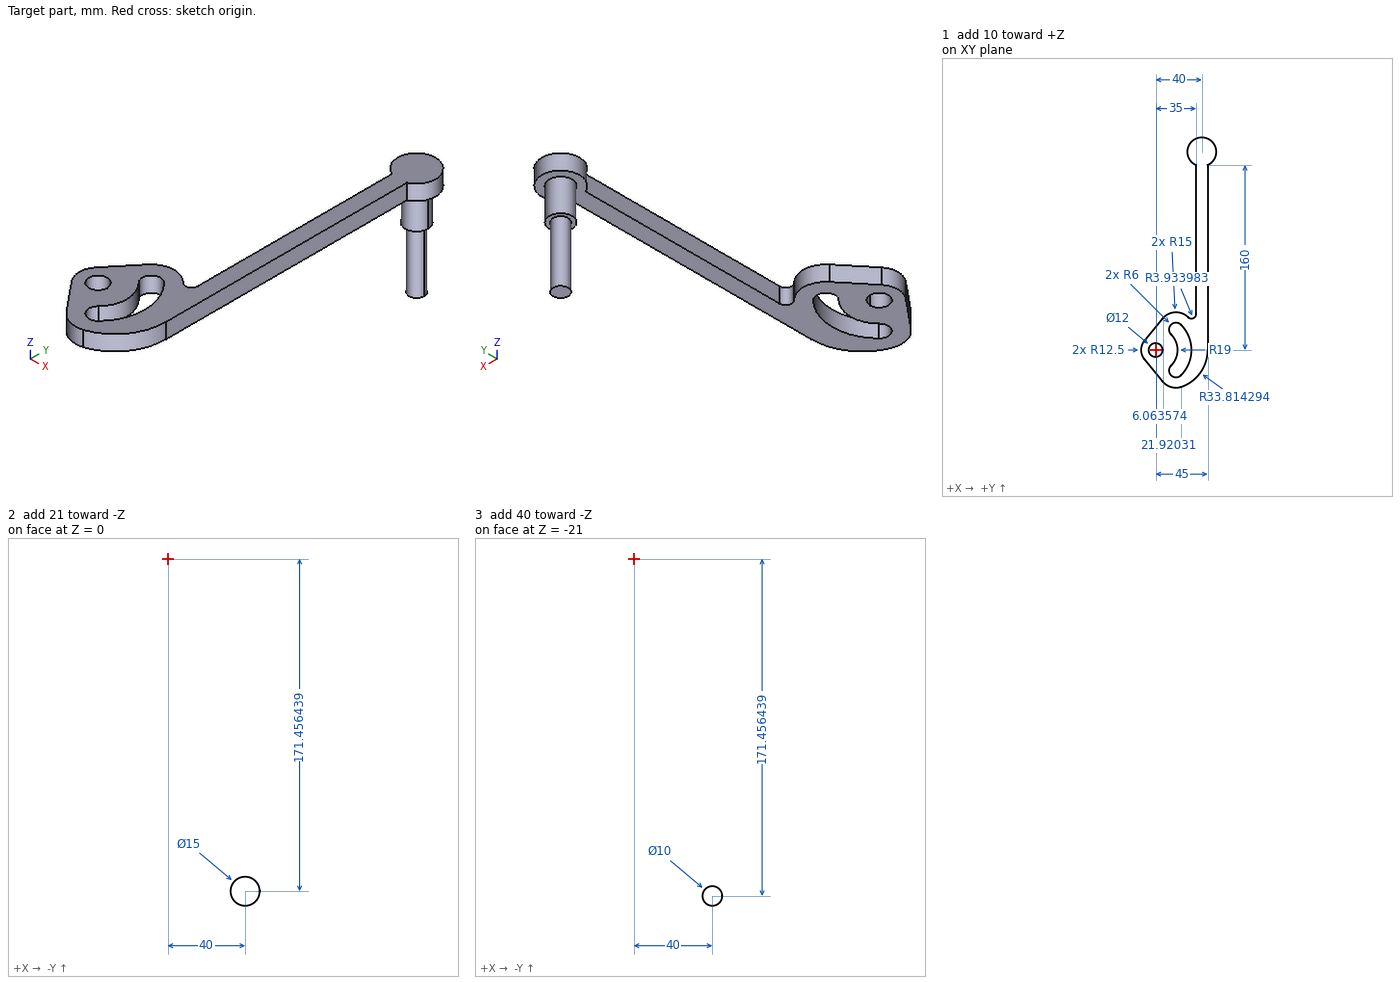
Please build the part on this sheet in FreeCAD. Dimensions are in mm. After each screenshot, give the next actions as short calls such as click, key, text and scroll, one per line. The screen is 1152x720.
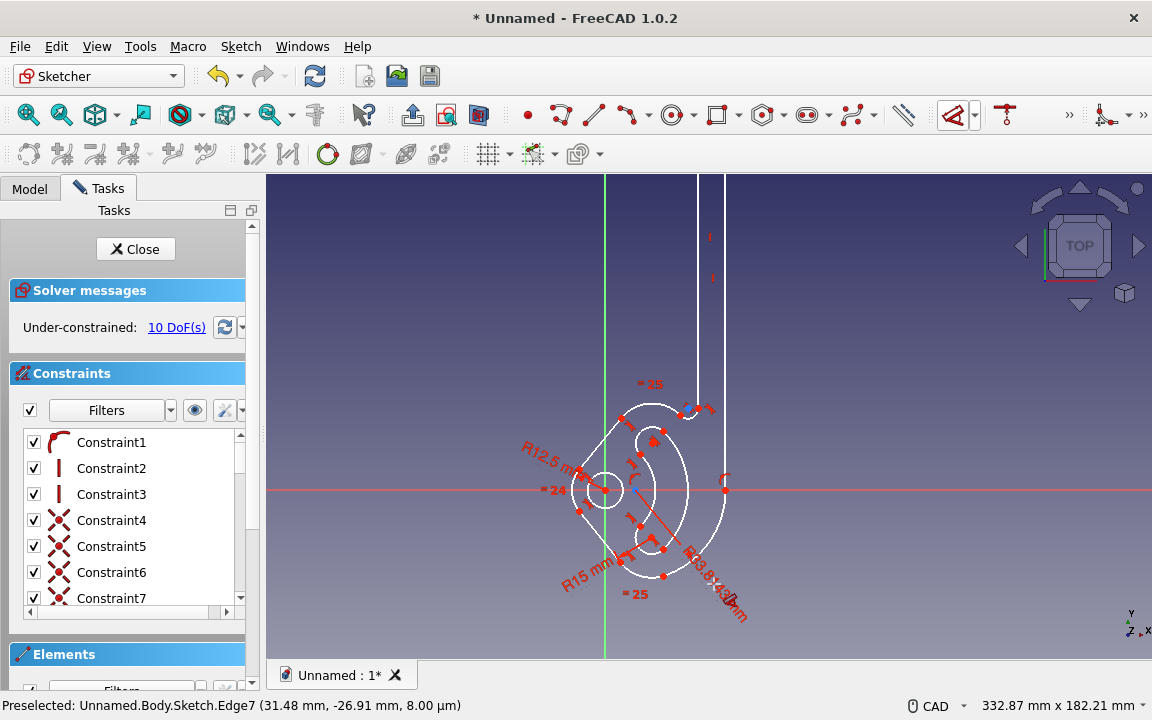
scroll(692, 418, up, 7)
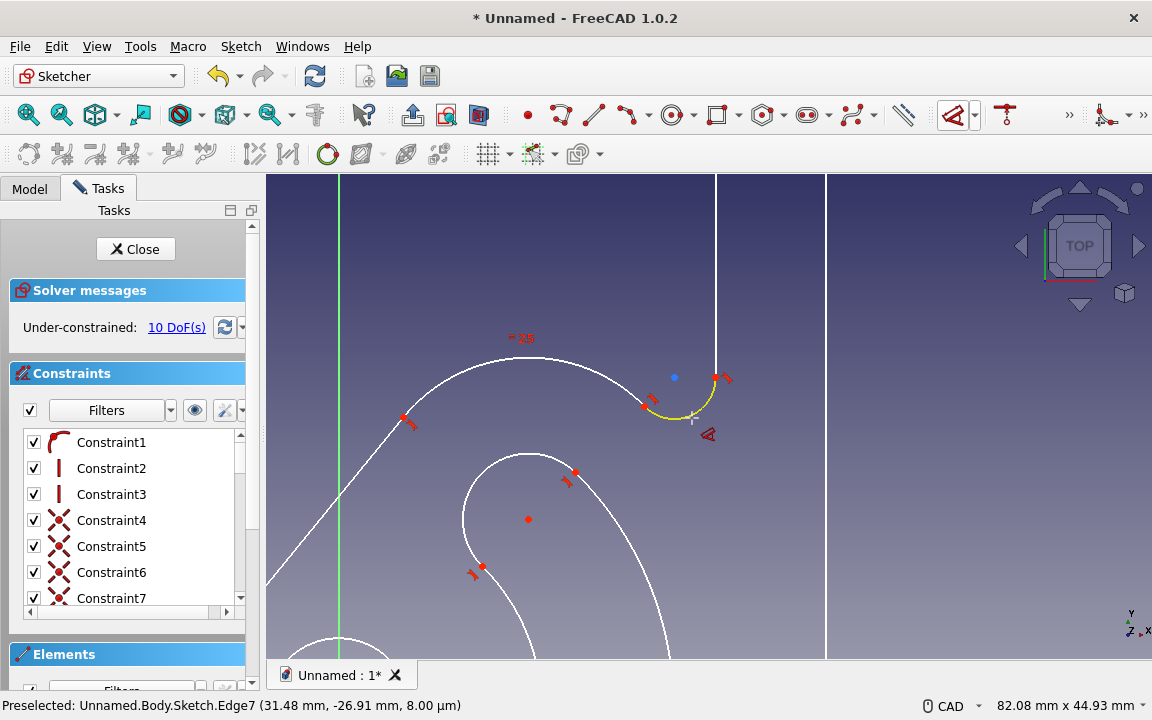
click(690, 416)
click(702, 446)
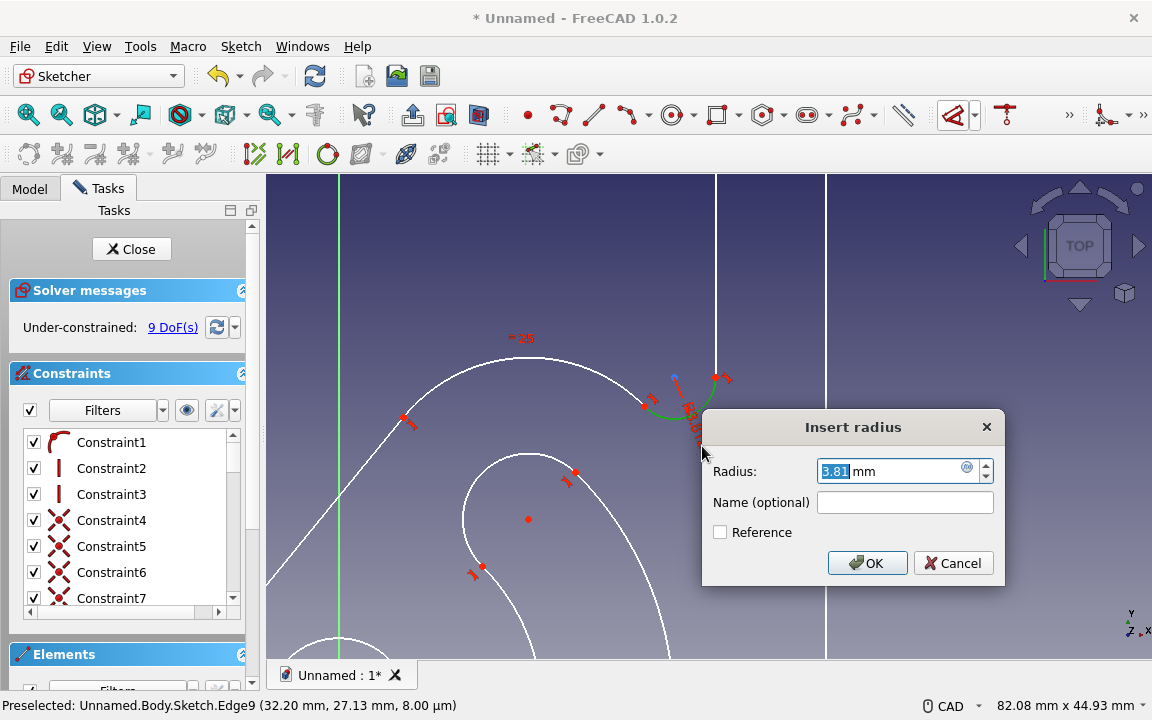
text(3.933983)
key(Return)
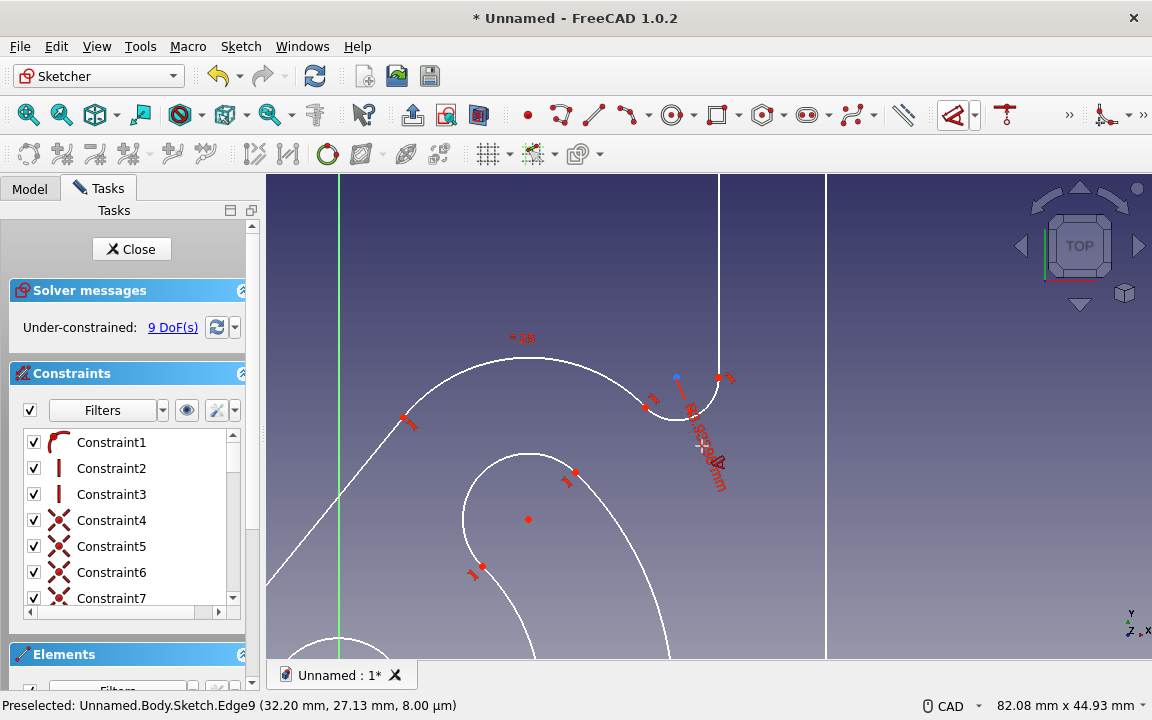
scroll(660, 499, down, 10)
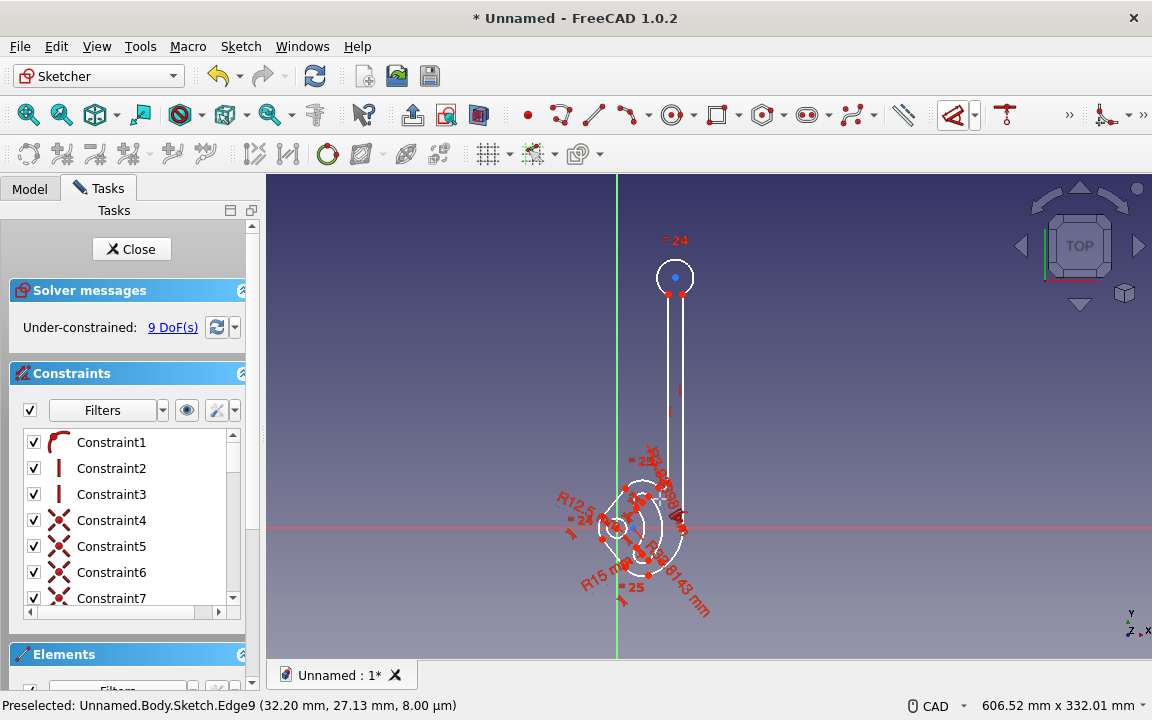
scroll(641, 516, up, 3)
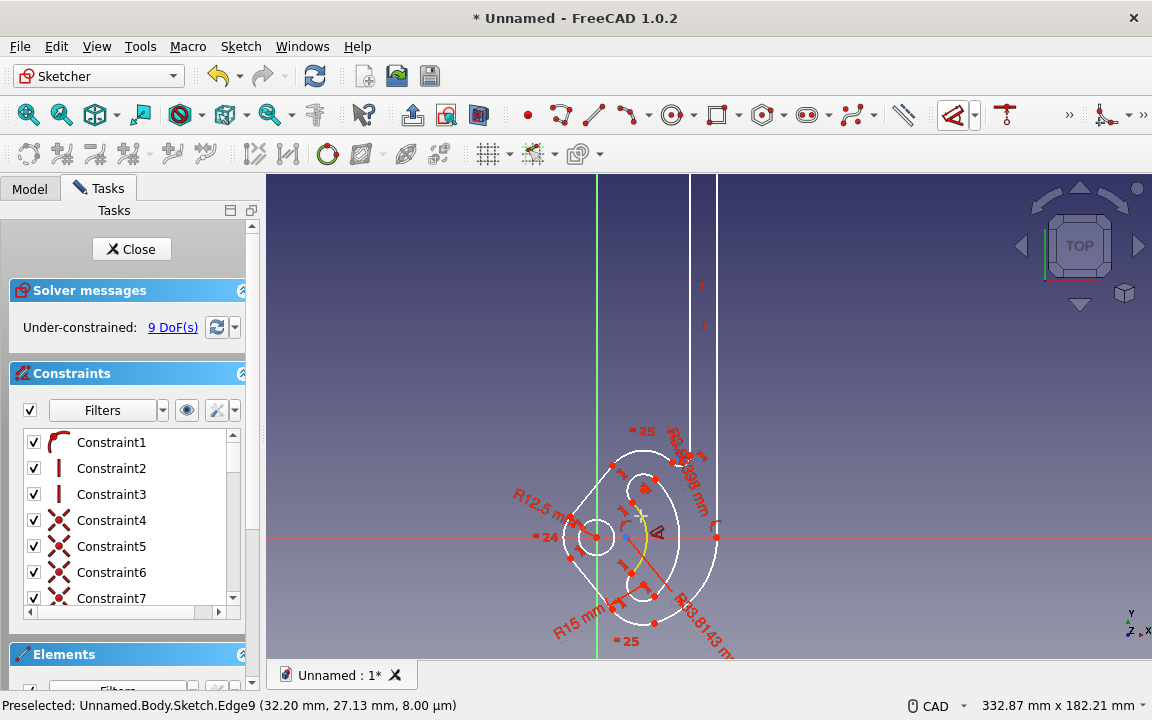
click(641, 515)
click(560, 465)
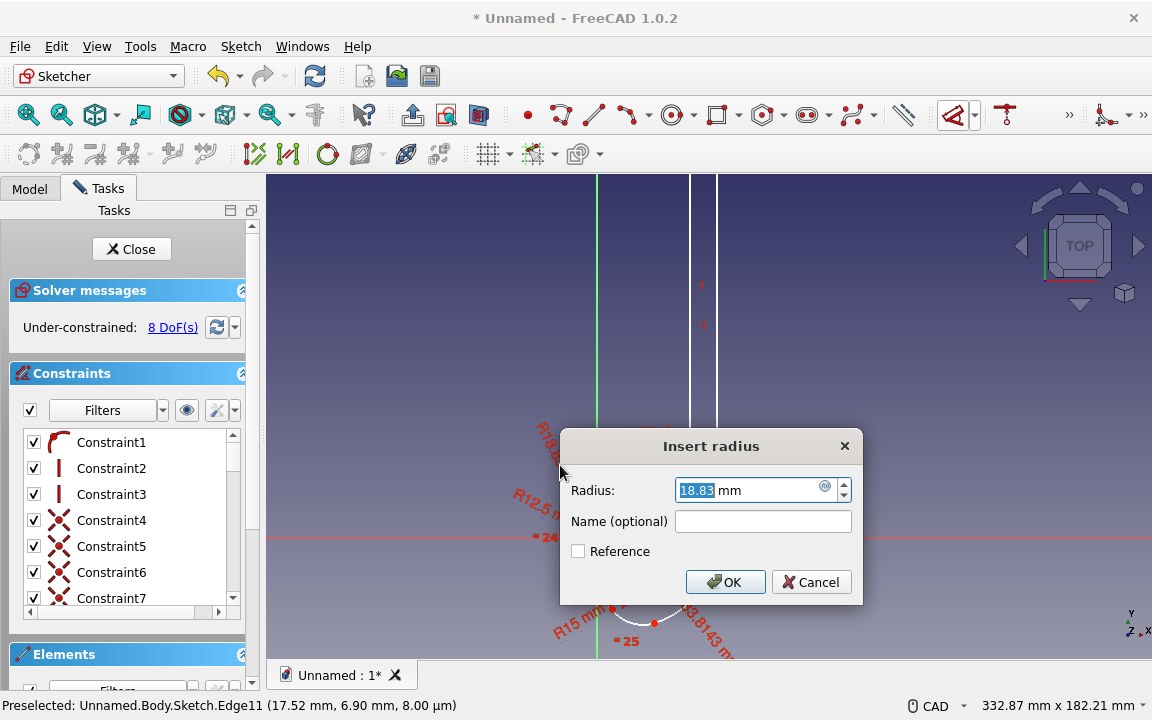
text(19)
key(Return)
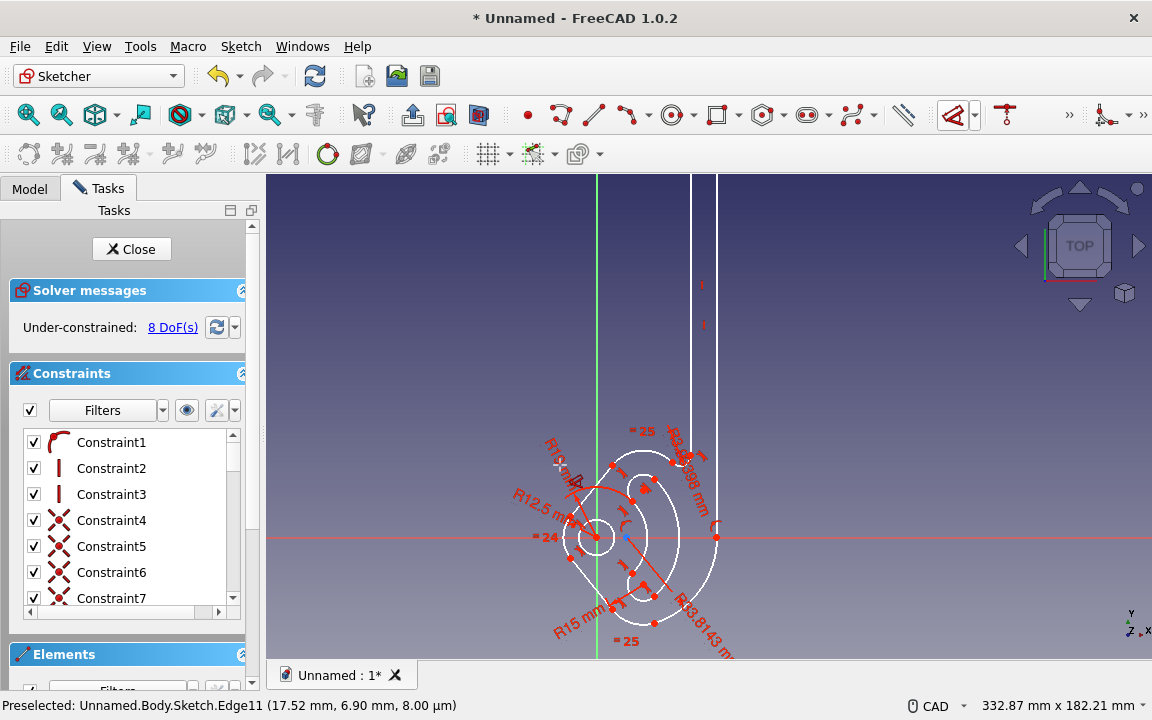
scroll(641, 475, up, 5)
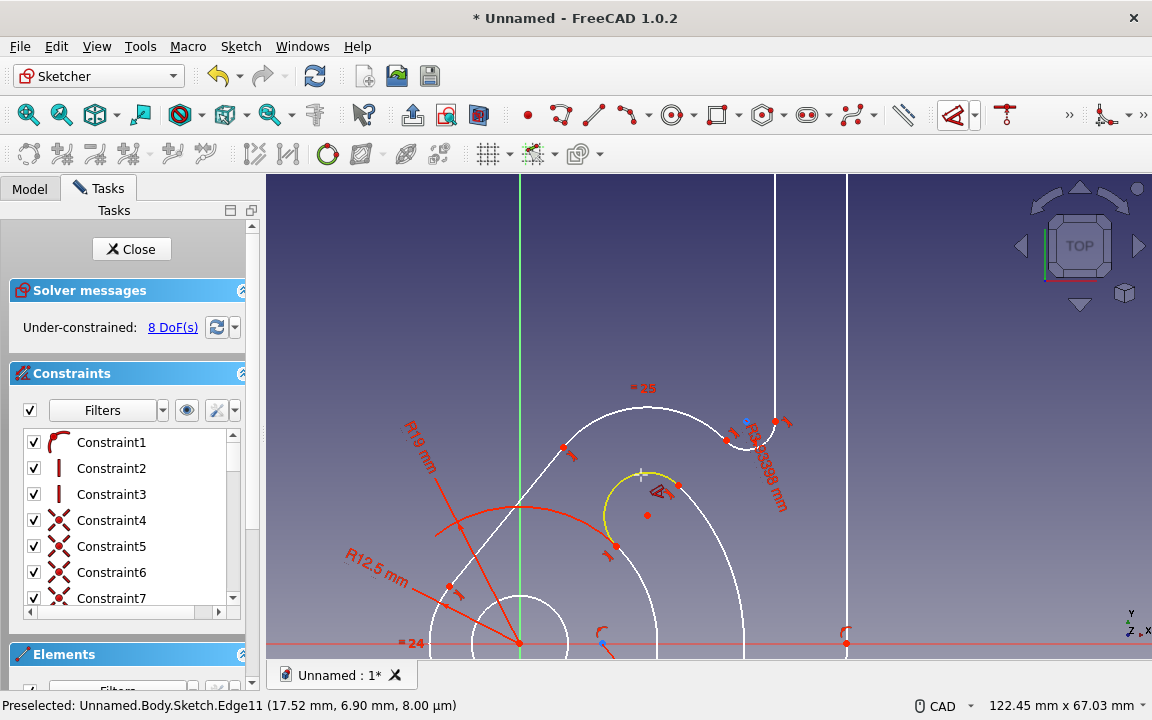
click(641, 473)
click(636, 441)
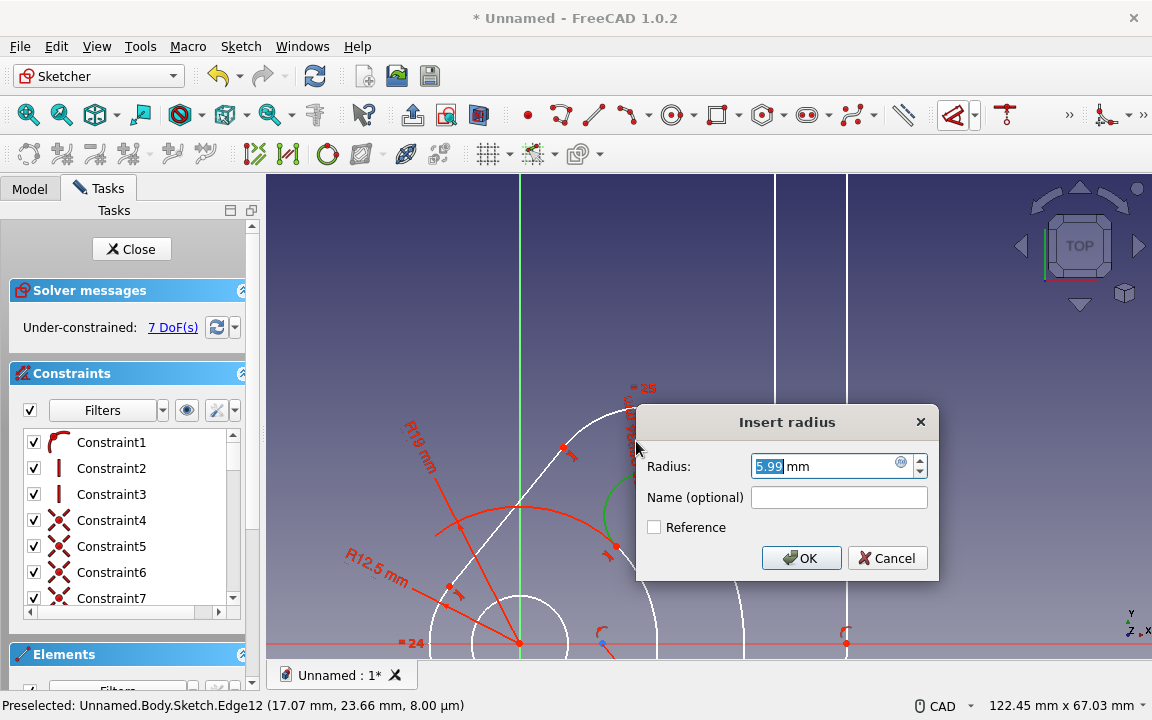
text(6)
key(Return)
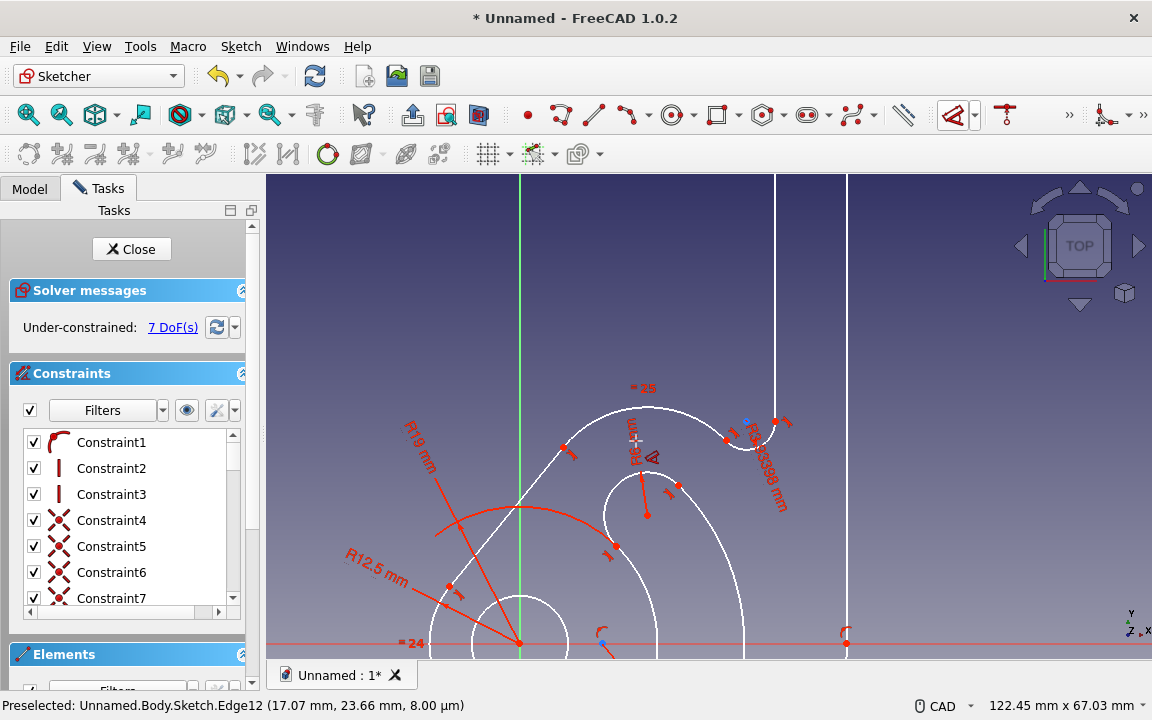
click(554, 610)
click(577, 587)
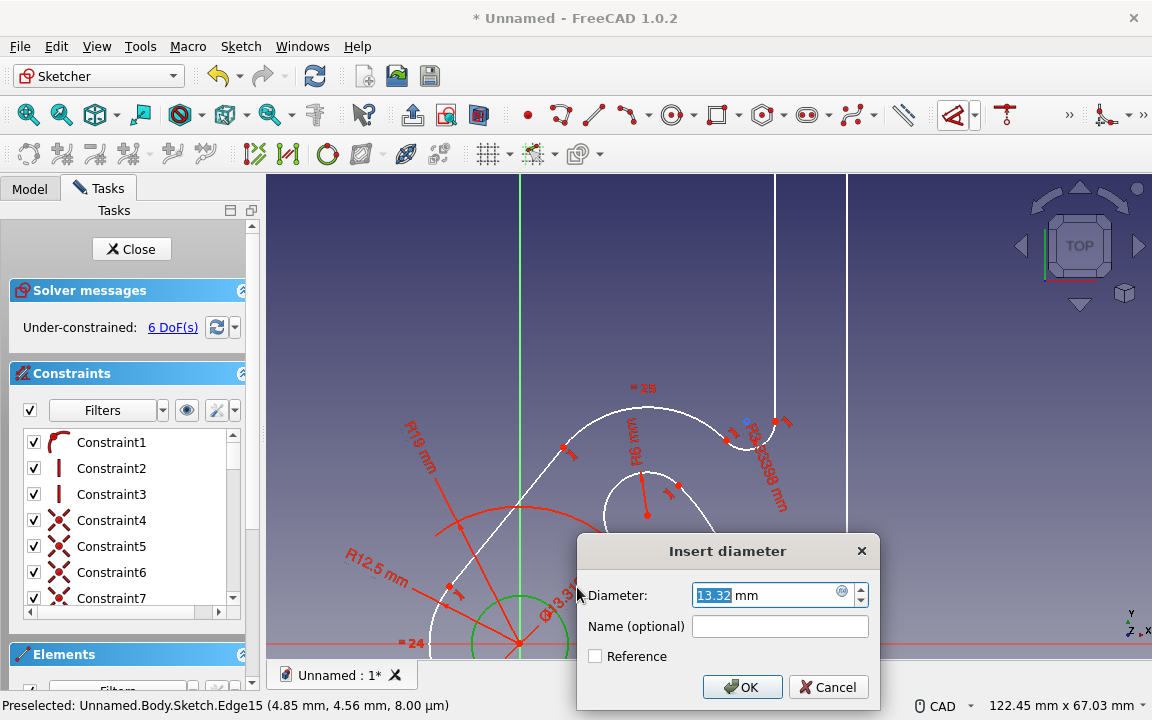
text(12)
key(Return)